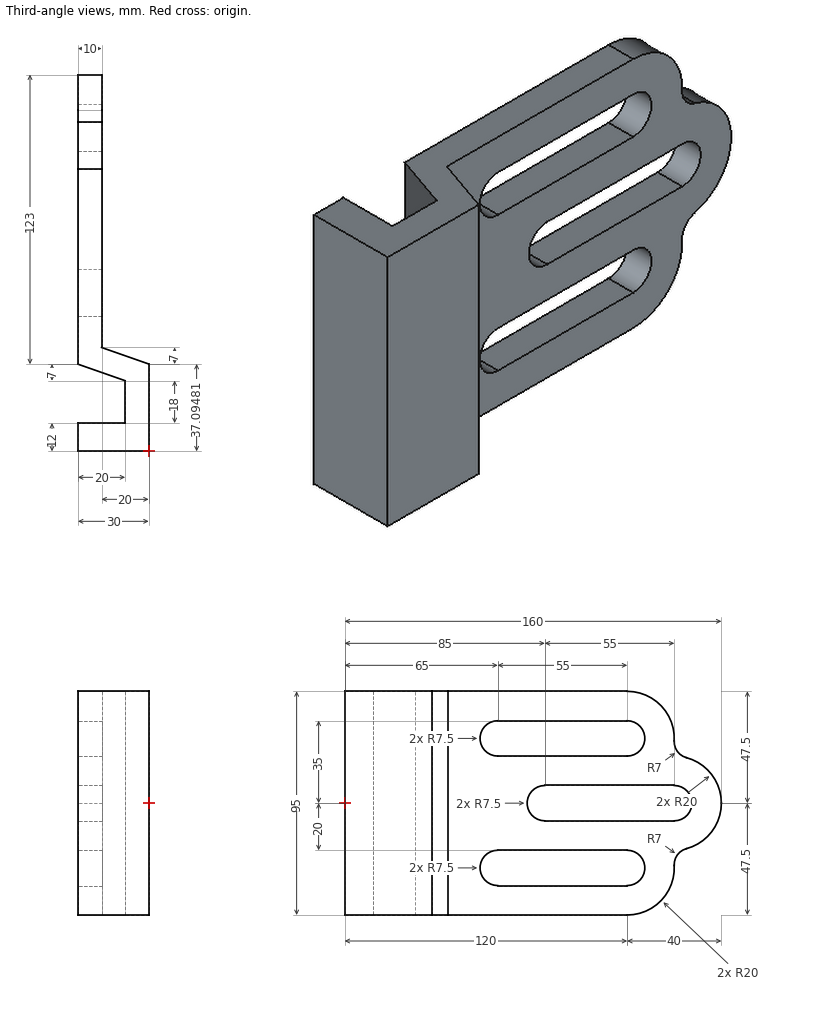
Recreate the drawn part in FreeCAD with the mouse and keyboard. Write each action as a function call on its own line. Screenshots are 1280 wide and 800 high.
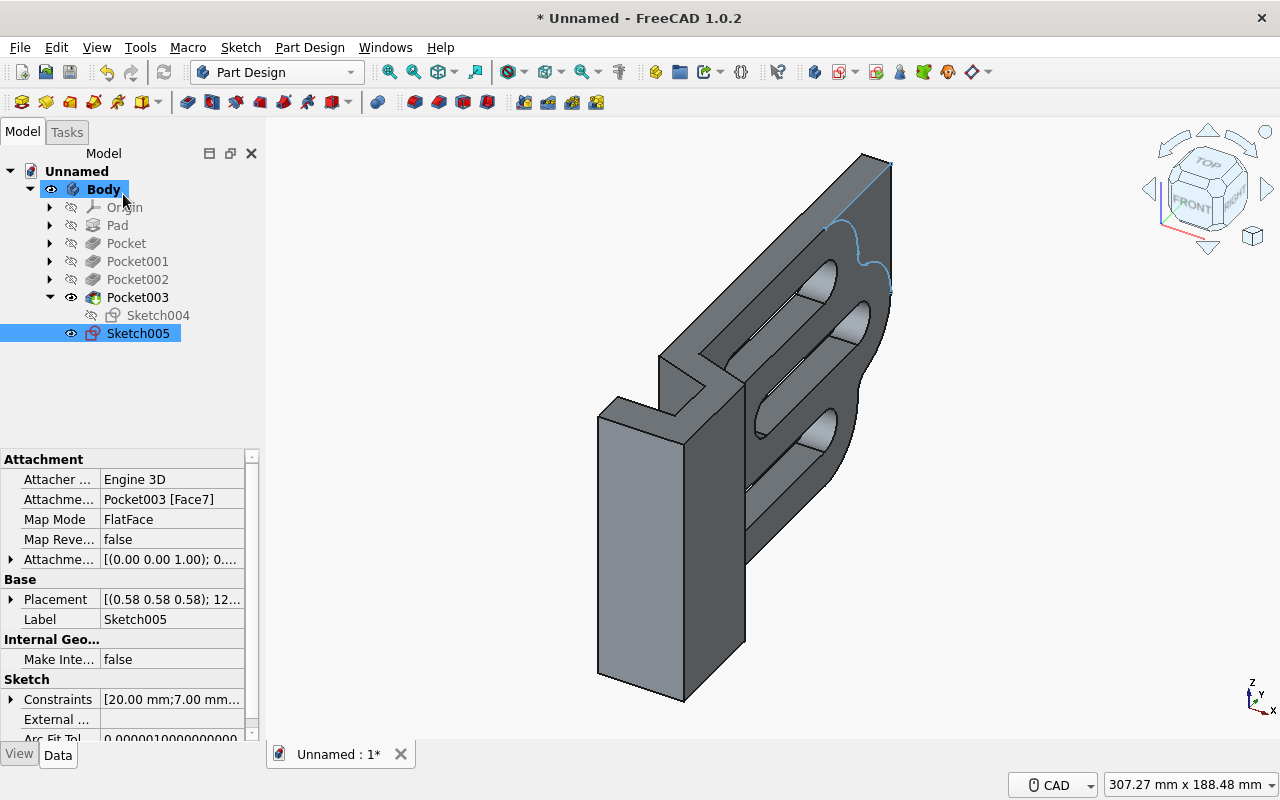
click(188, 102)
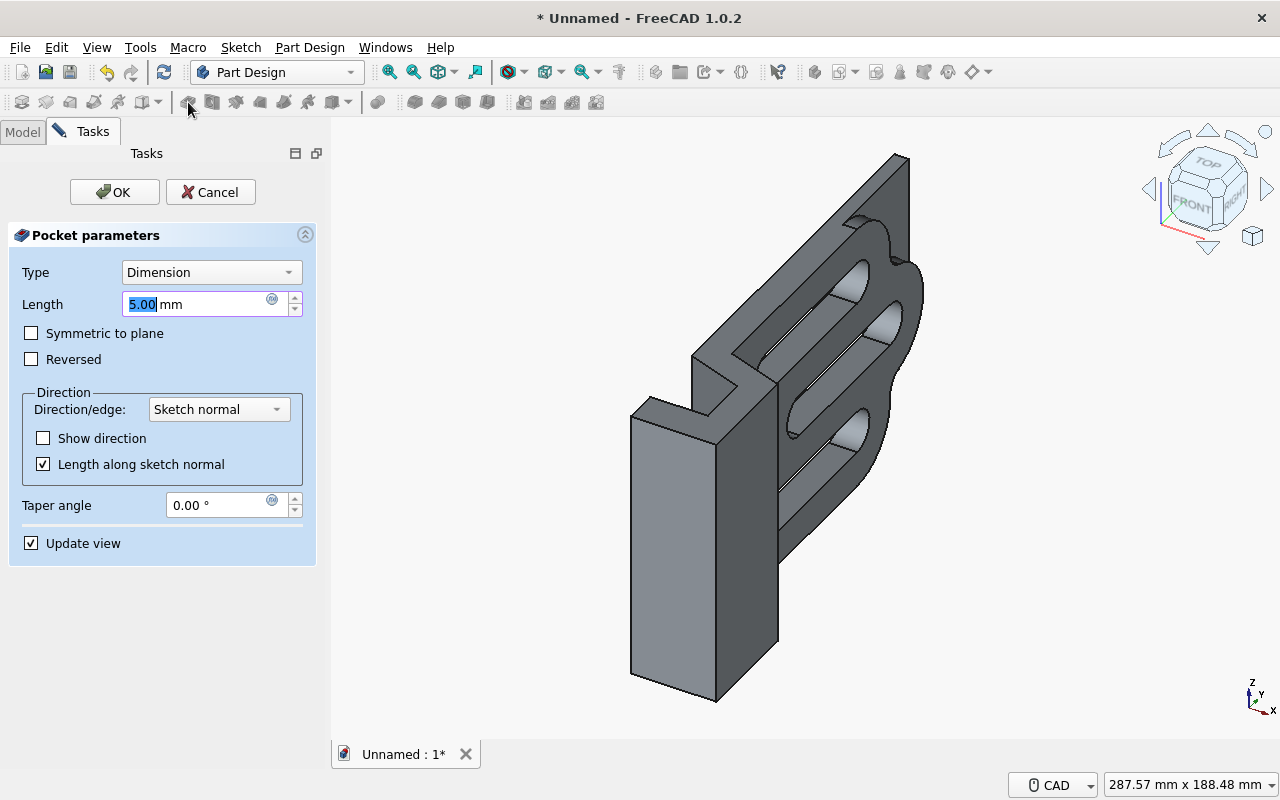
click(212, 272)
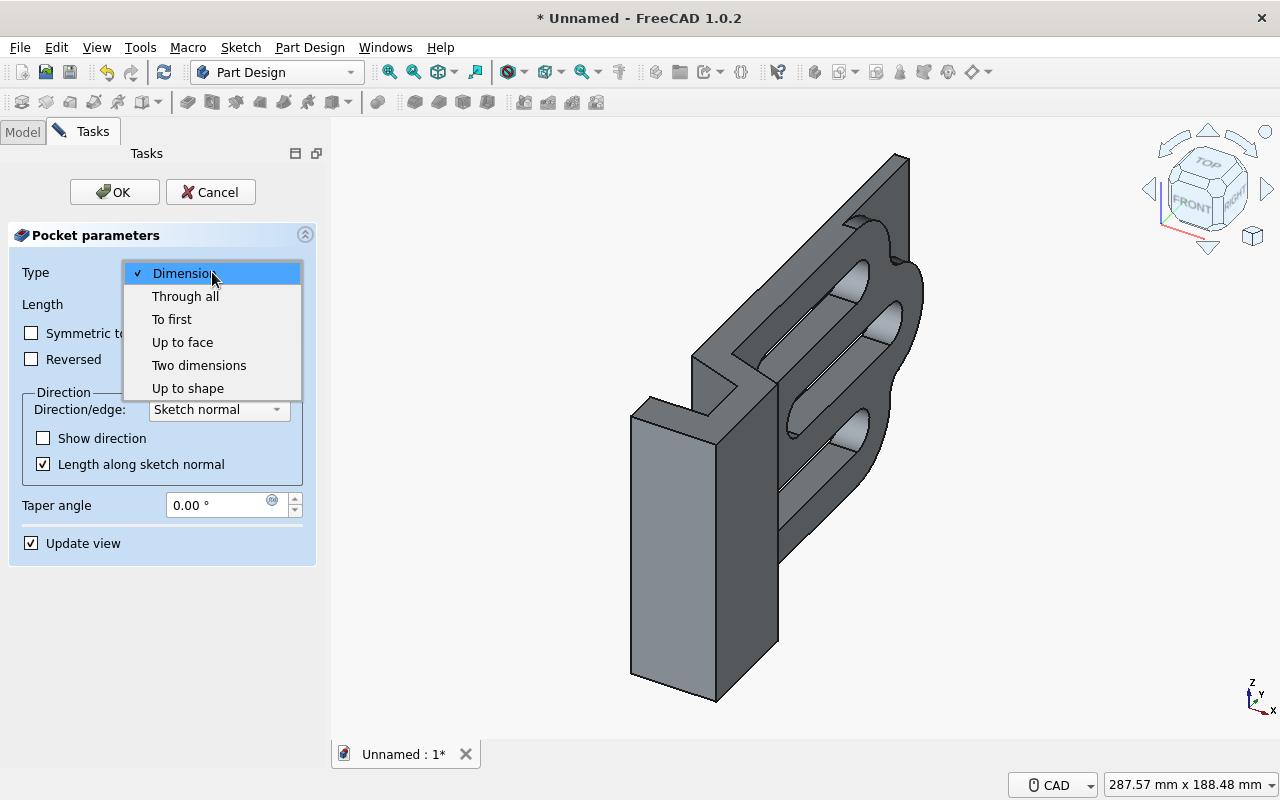
click(212, 320)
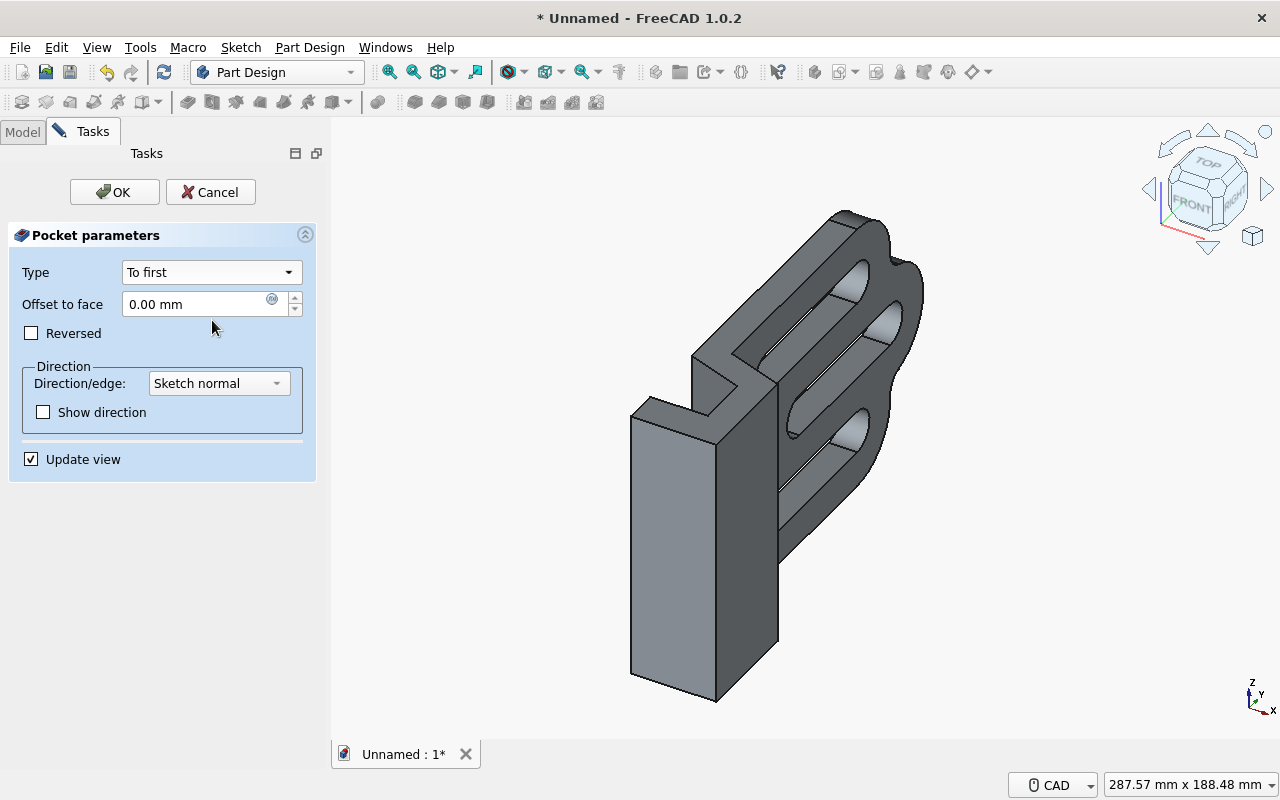
click(115, 192)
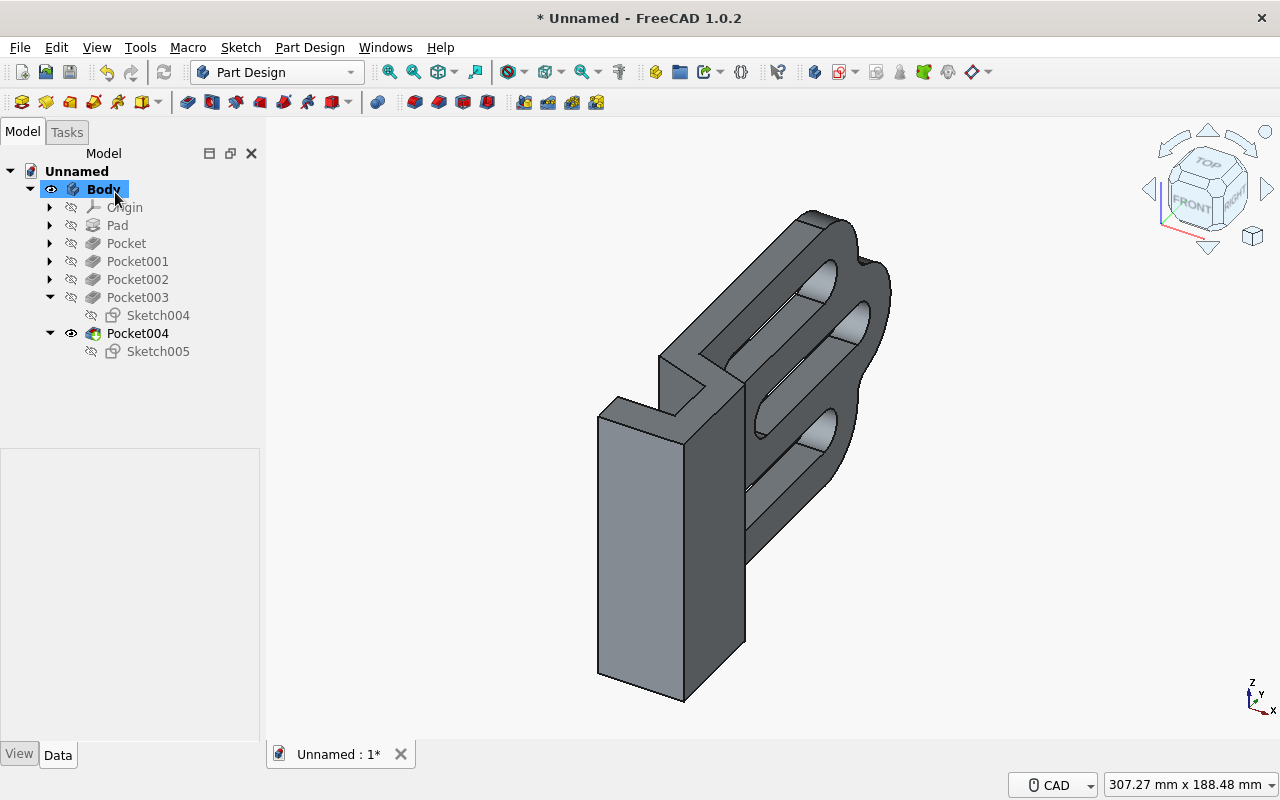
key(0)